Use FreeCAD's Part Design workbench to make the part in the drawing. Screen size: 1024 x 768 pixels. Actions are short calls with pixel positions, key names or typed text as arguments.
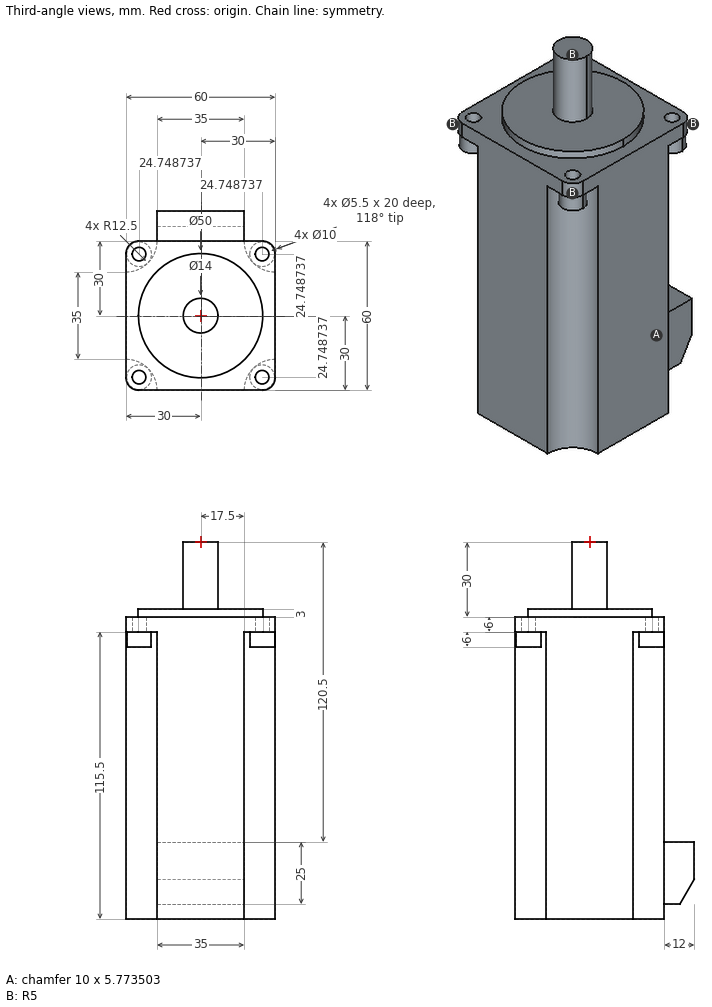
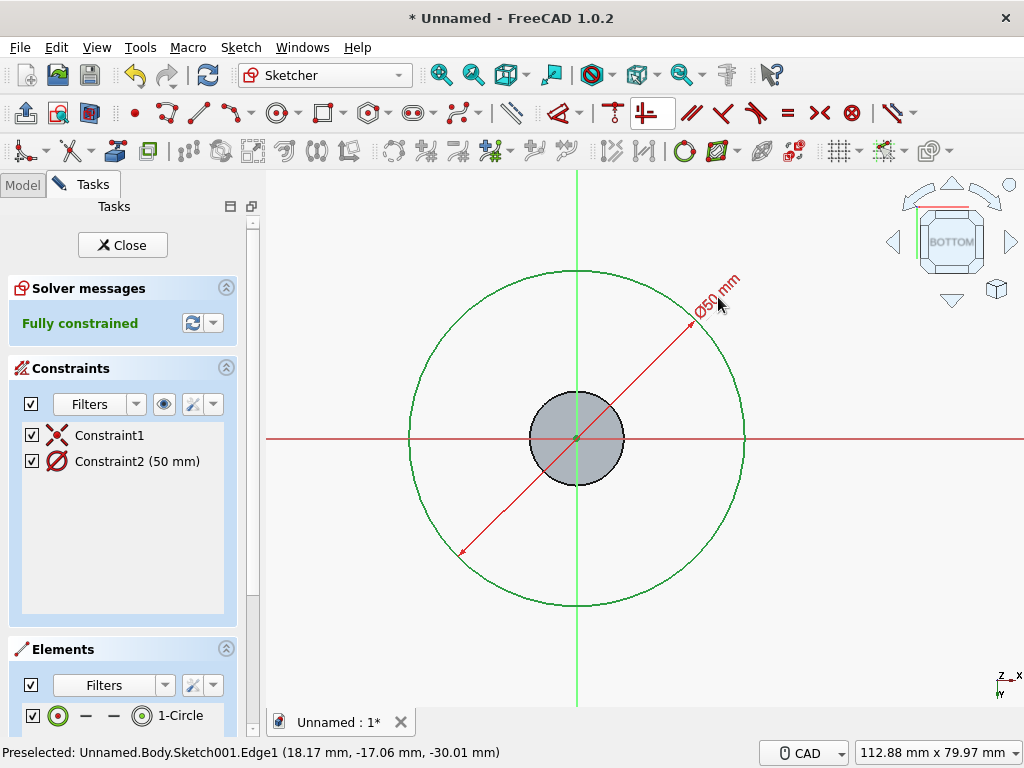
click(123, 245)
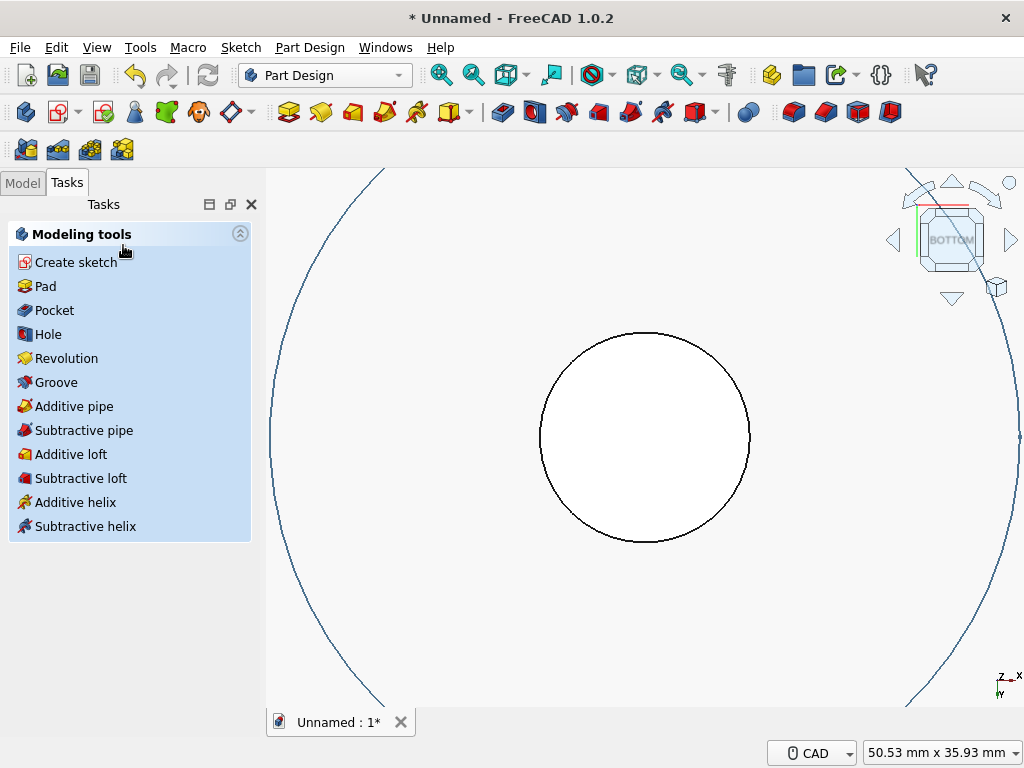
click(290, 112)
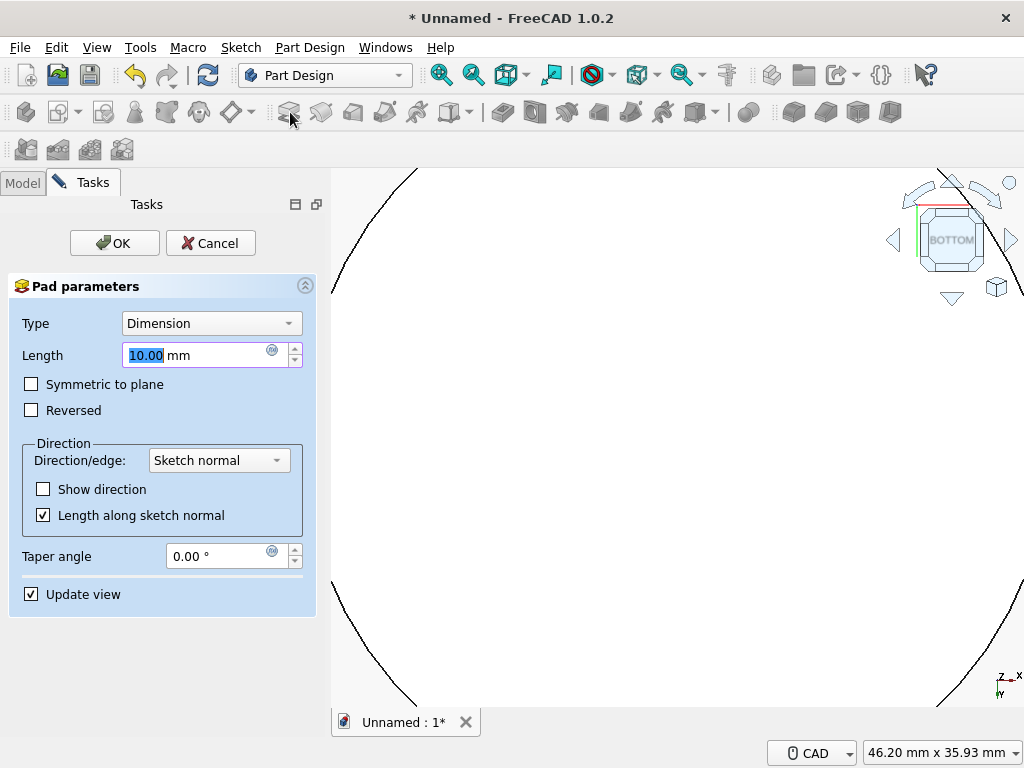
text(3)
key(Tab)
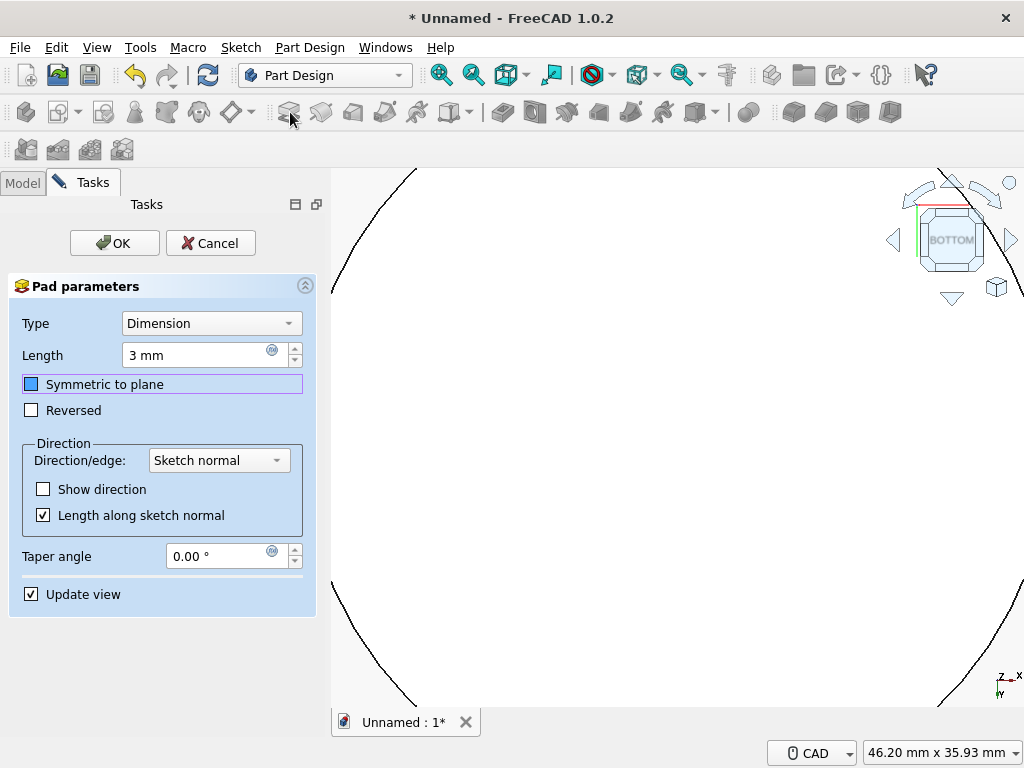
click(30, 410)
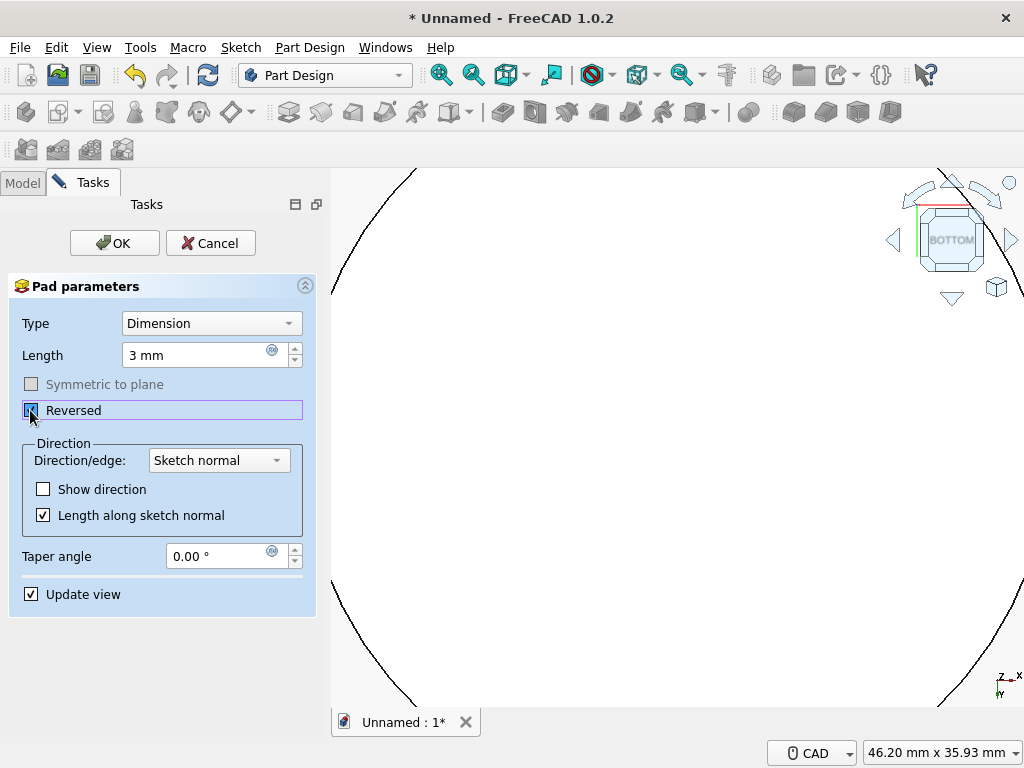
click(115, 243)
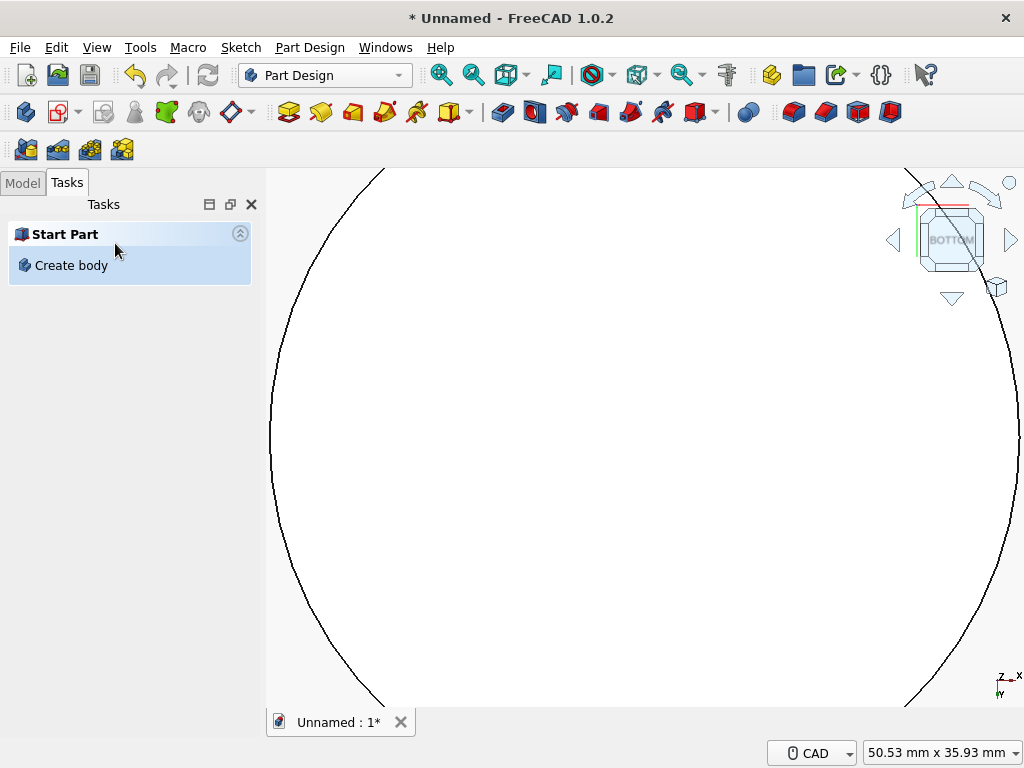
click(442, 76)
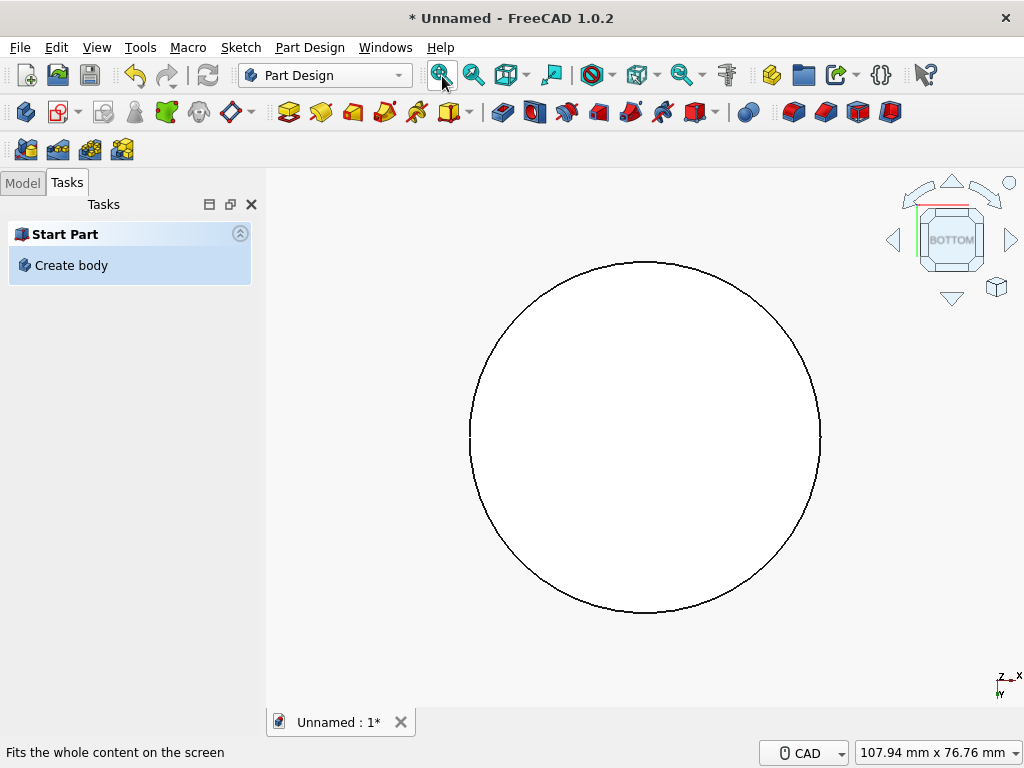
click(645, 436)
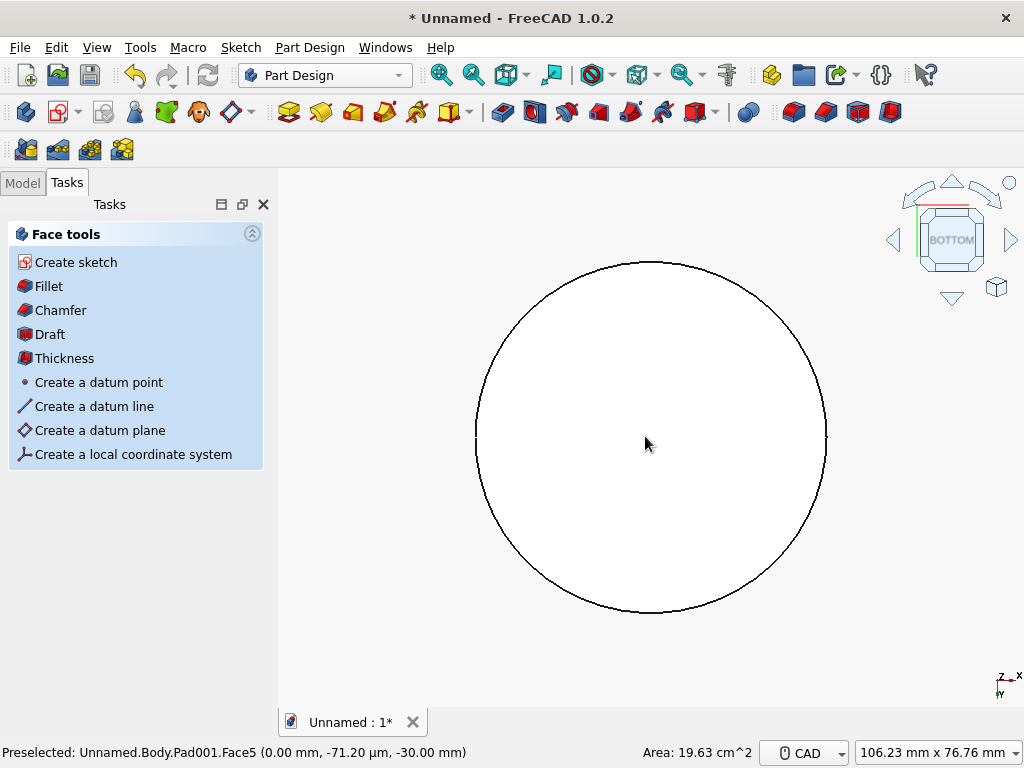
click(58, 112)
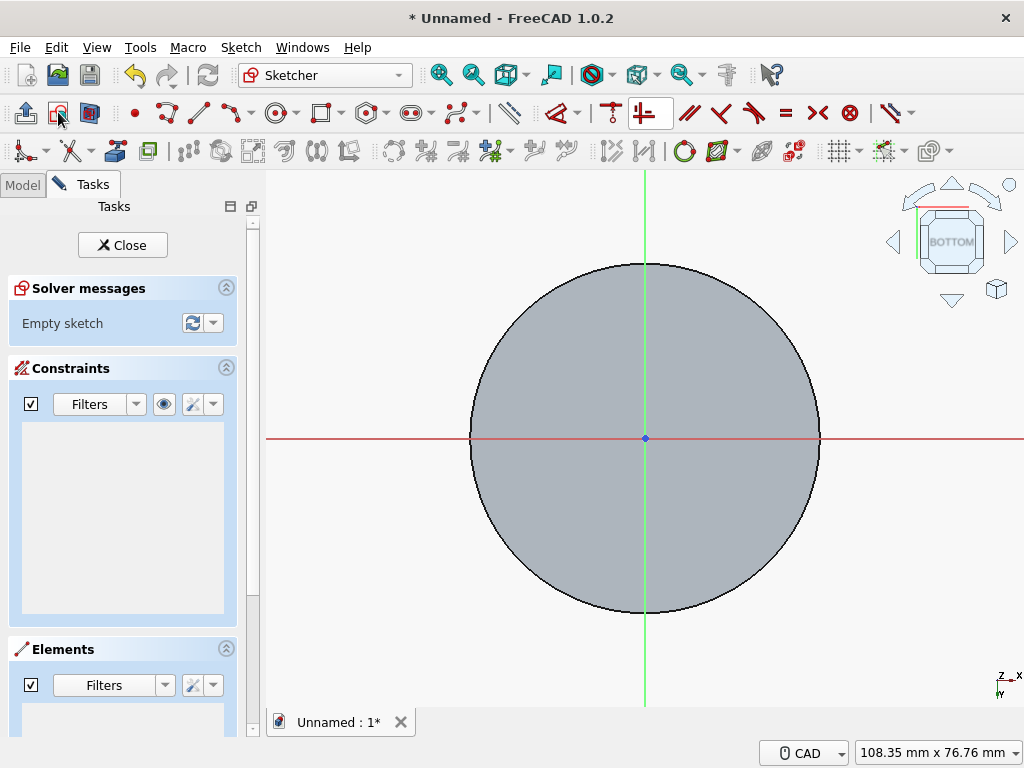
scroll(294, 439, down, 1)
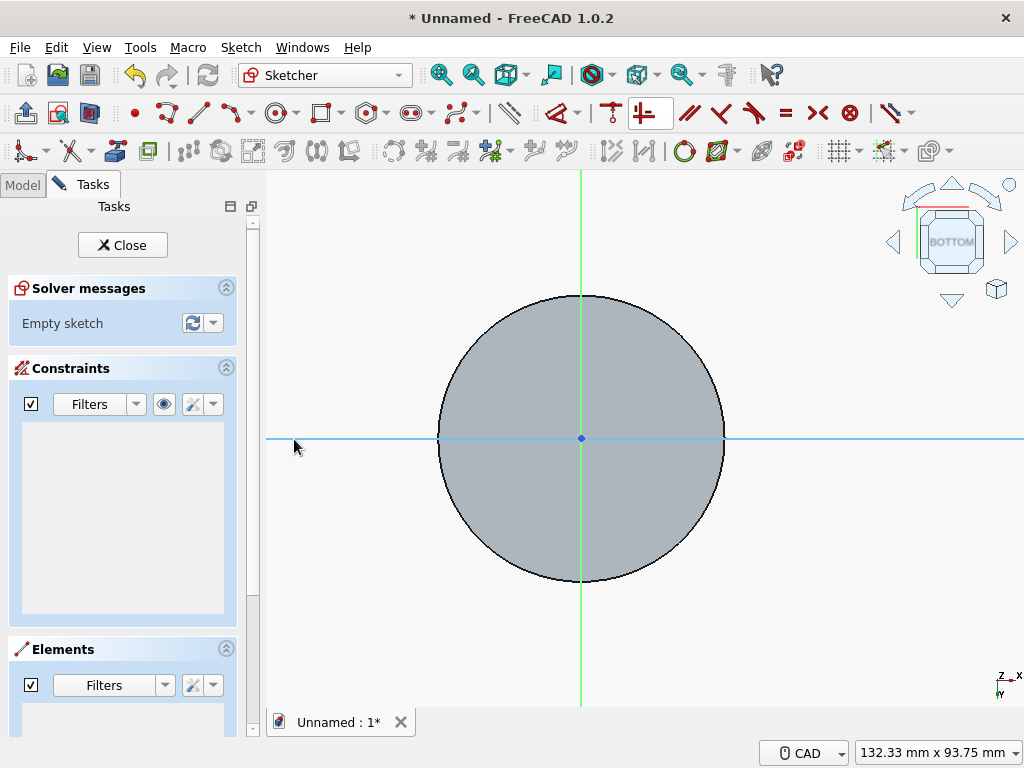
key(g)
key(v)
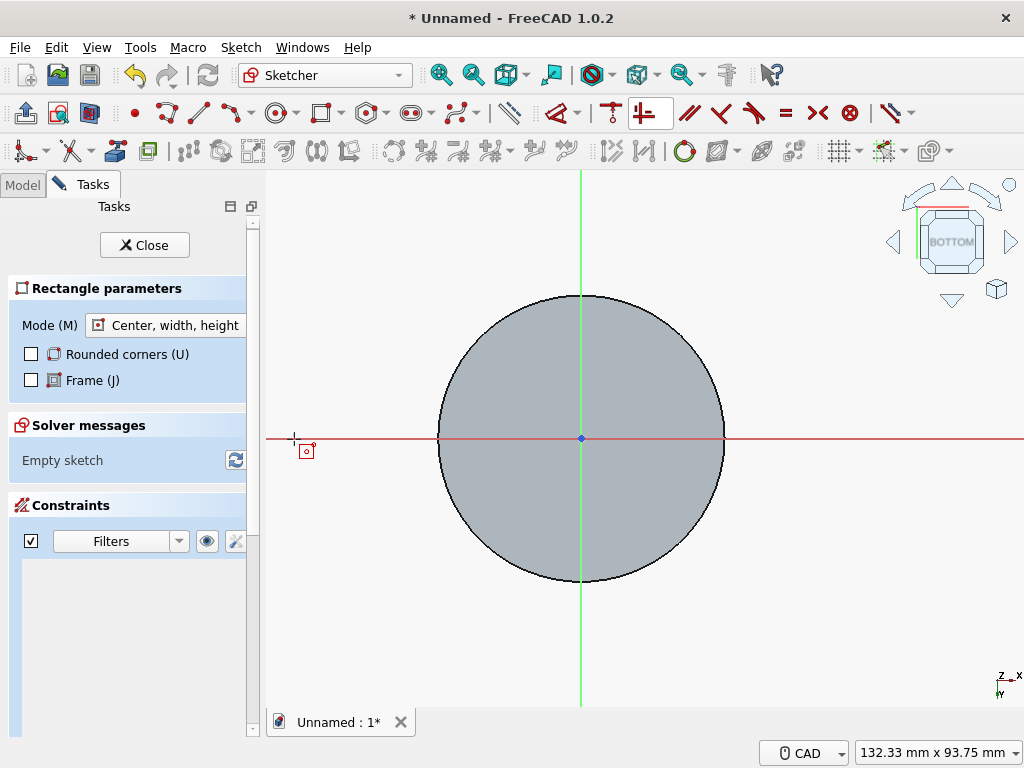
click(581, 439)
click(753, 267)
key(Escape)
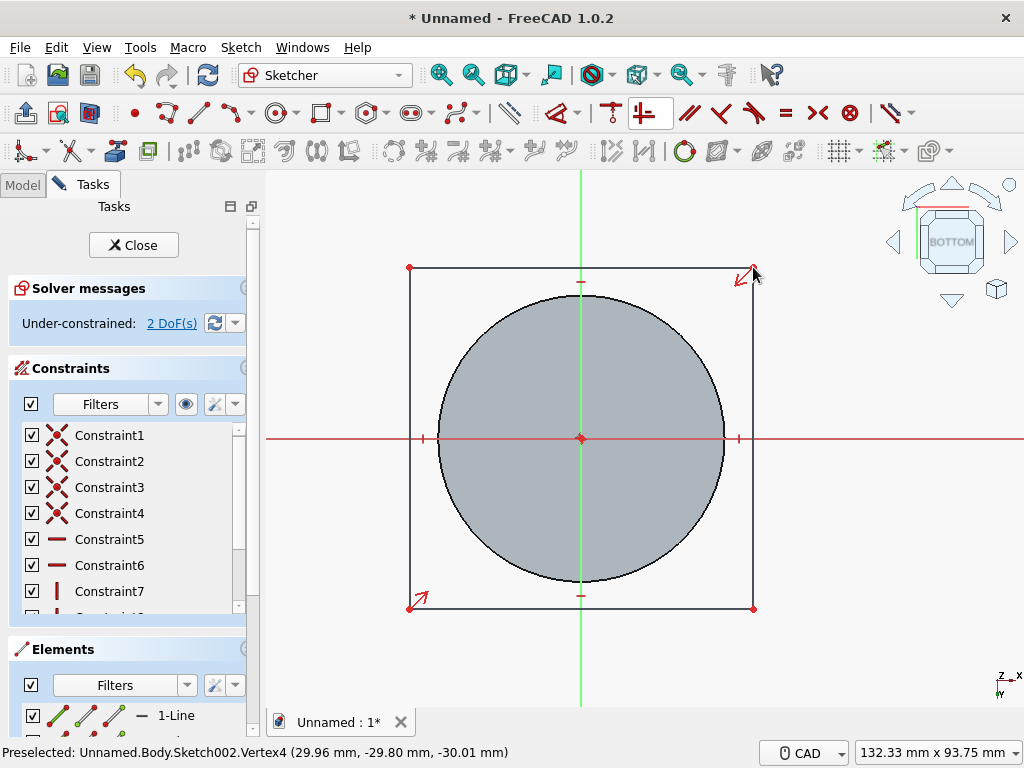
click(556, 114)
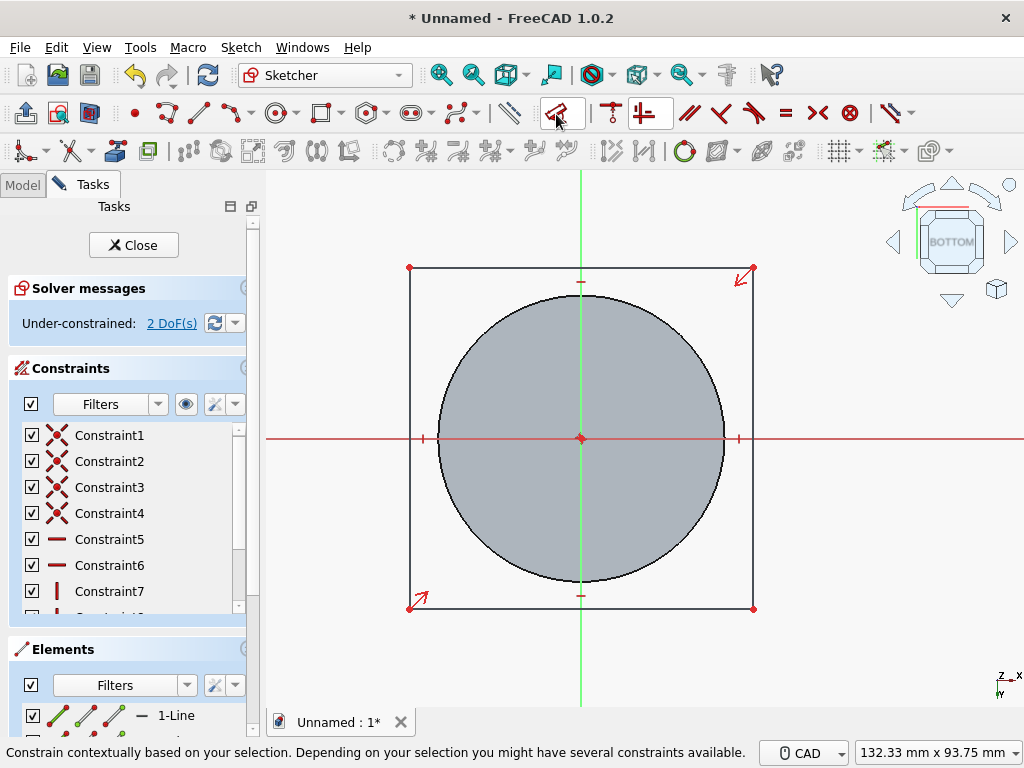
click(513, 609)
click(502, 643)